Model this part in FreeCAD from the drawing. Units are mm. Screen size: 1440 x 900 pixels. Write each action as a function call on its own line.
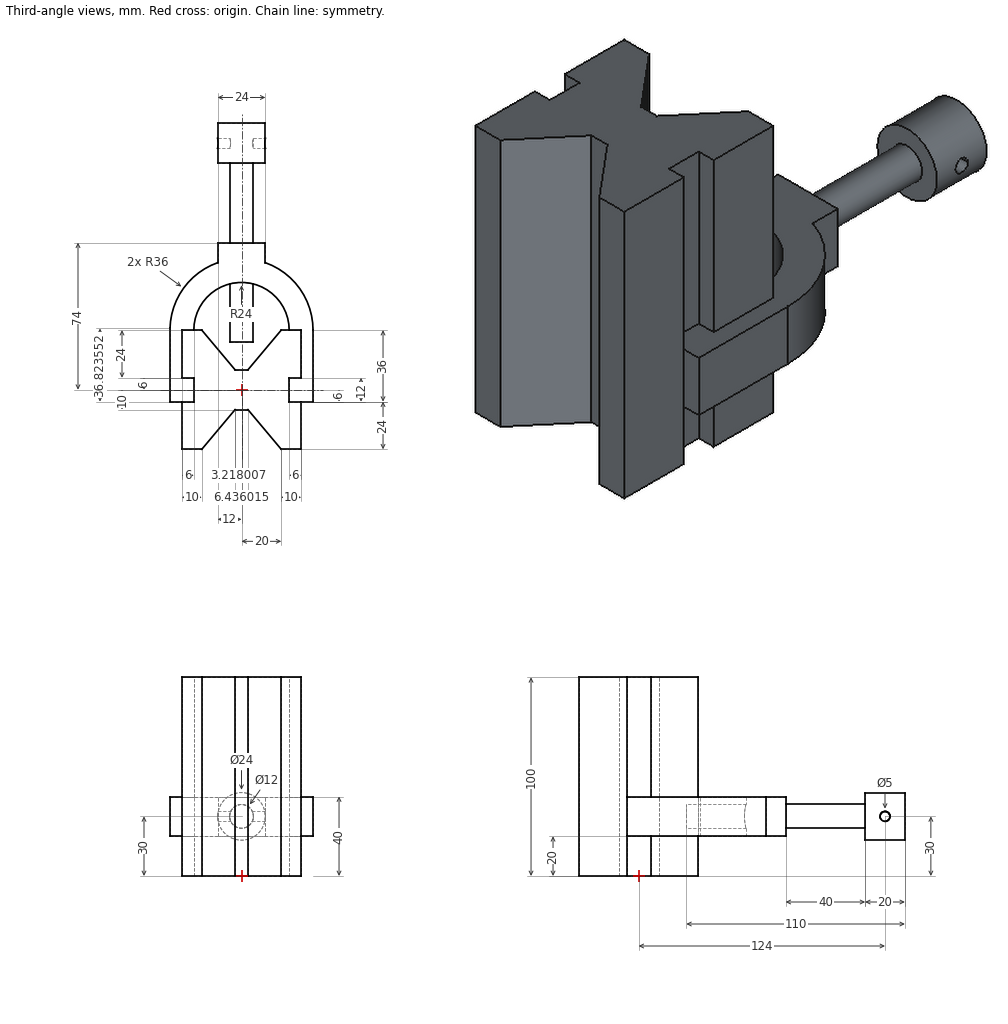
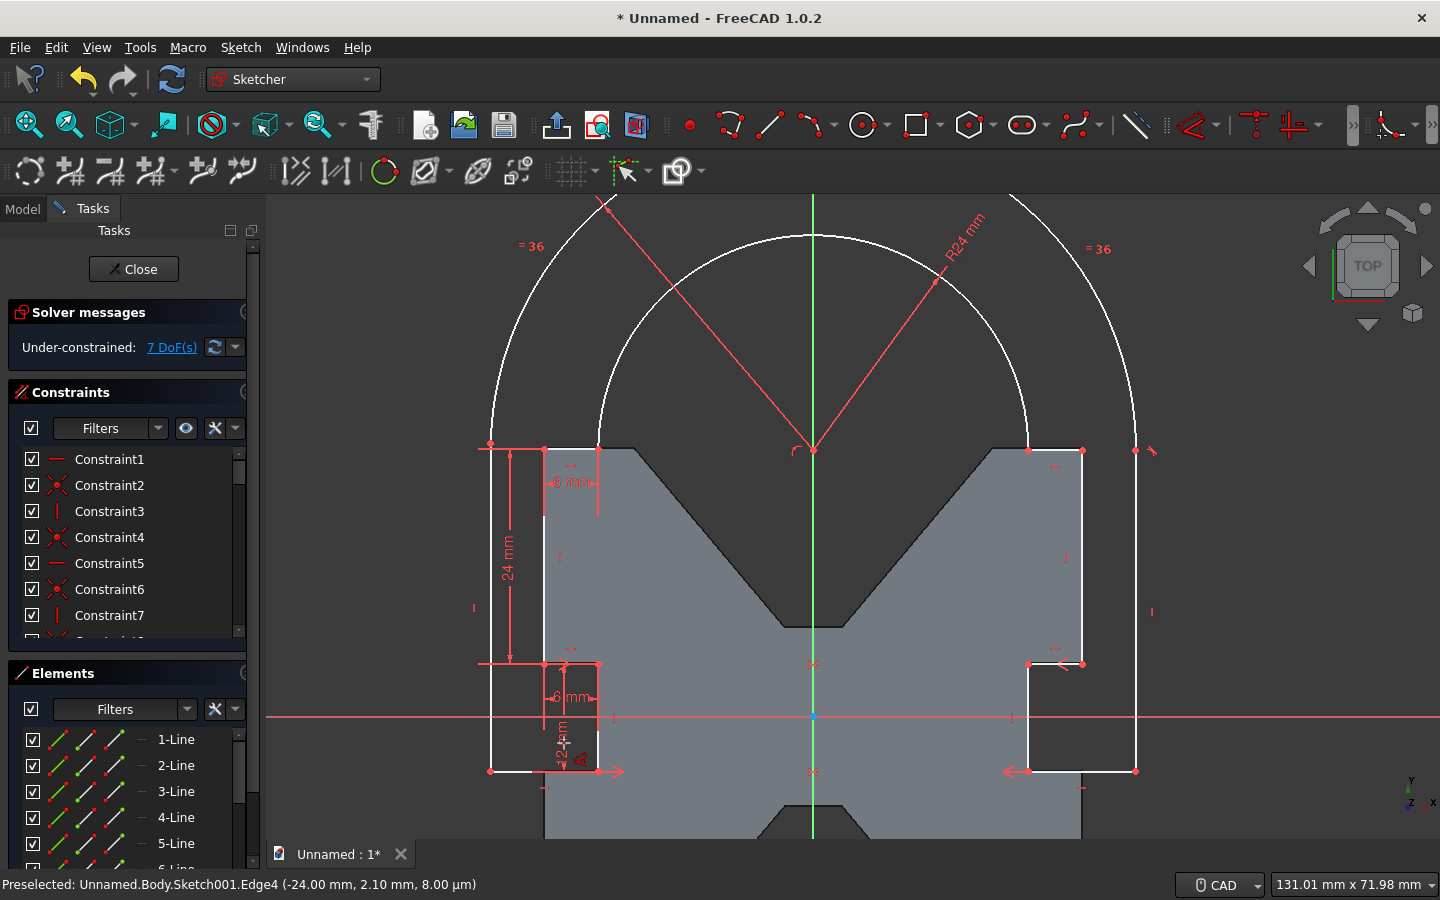
scroll(749, 643, down, 3)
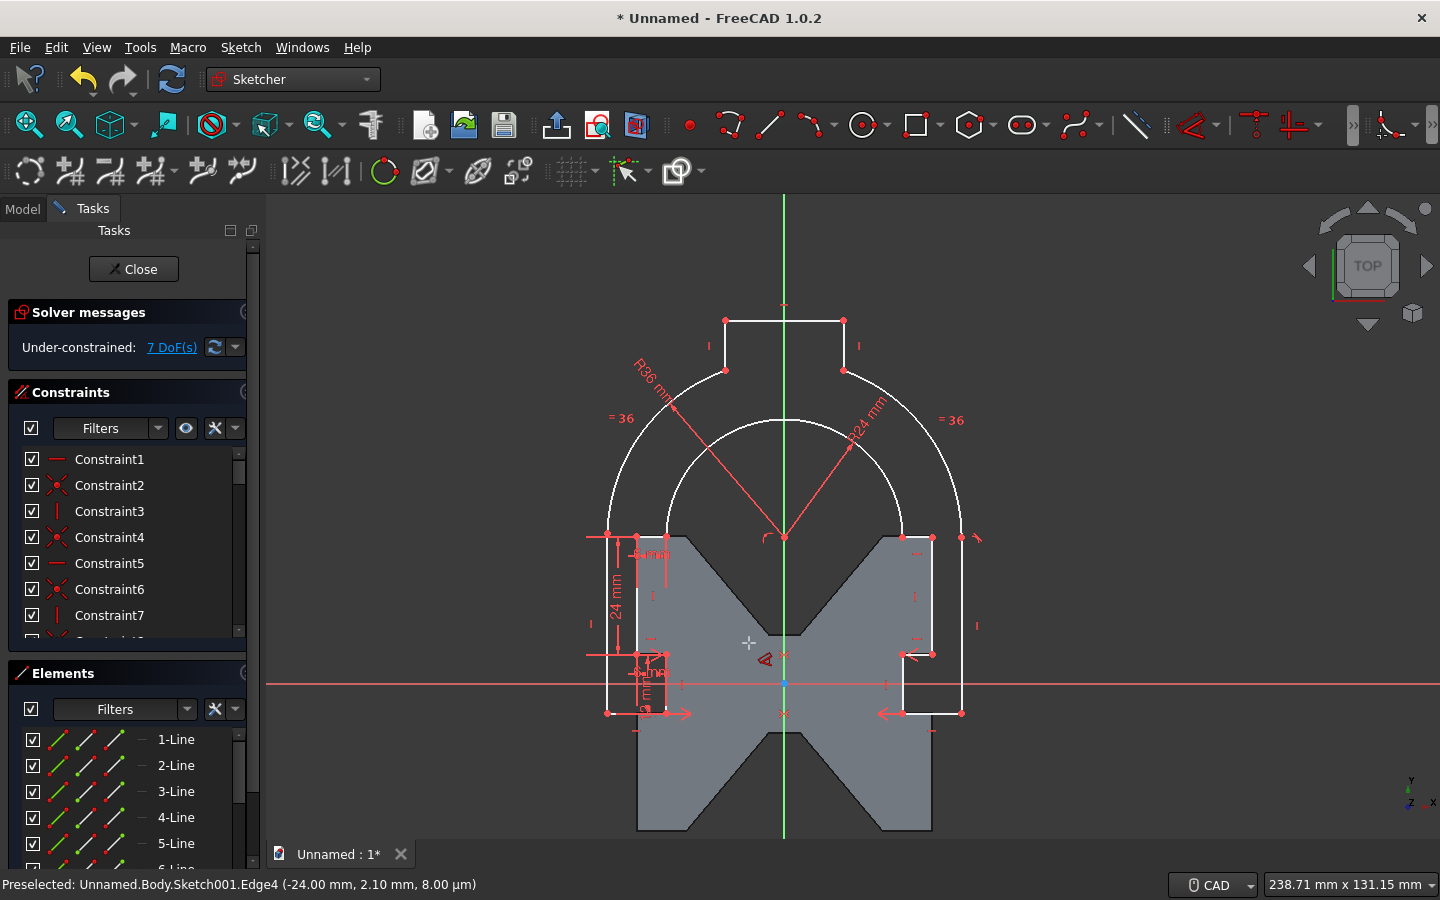
click(761, 321)
click(757, 287)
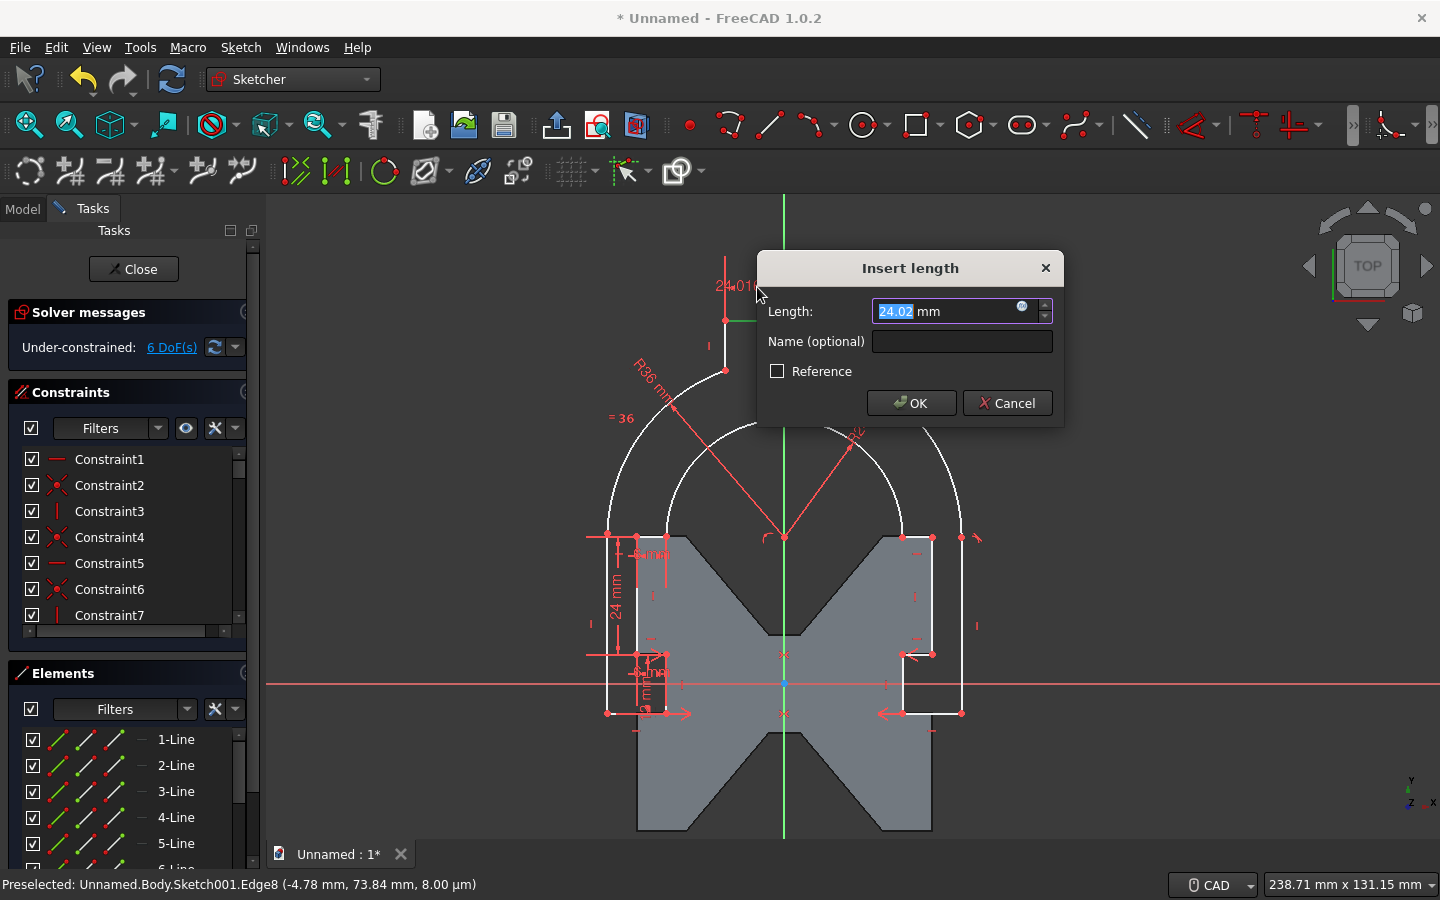
text(24)
key(Return)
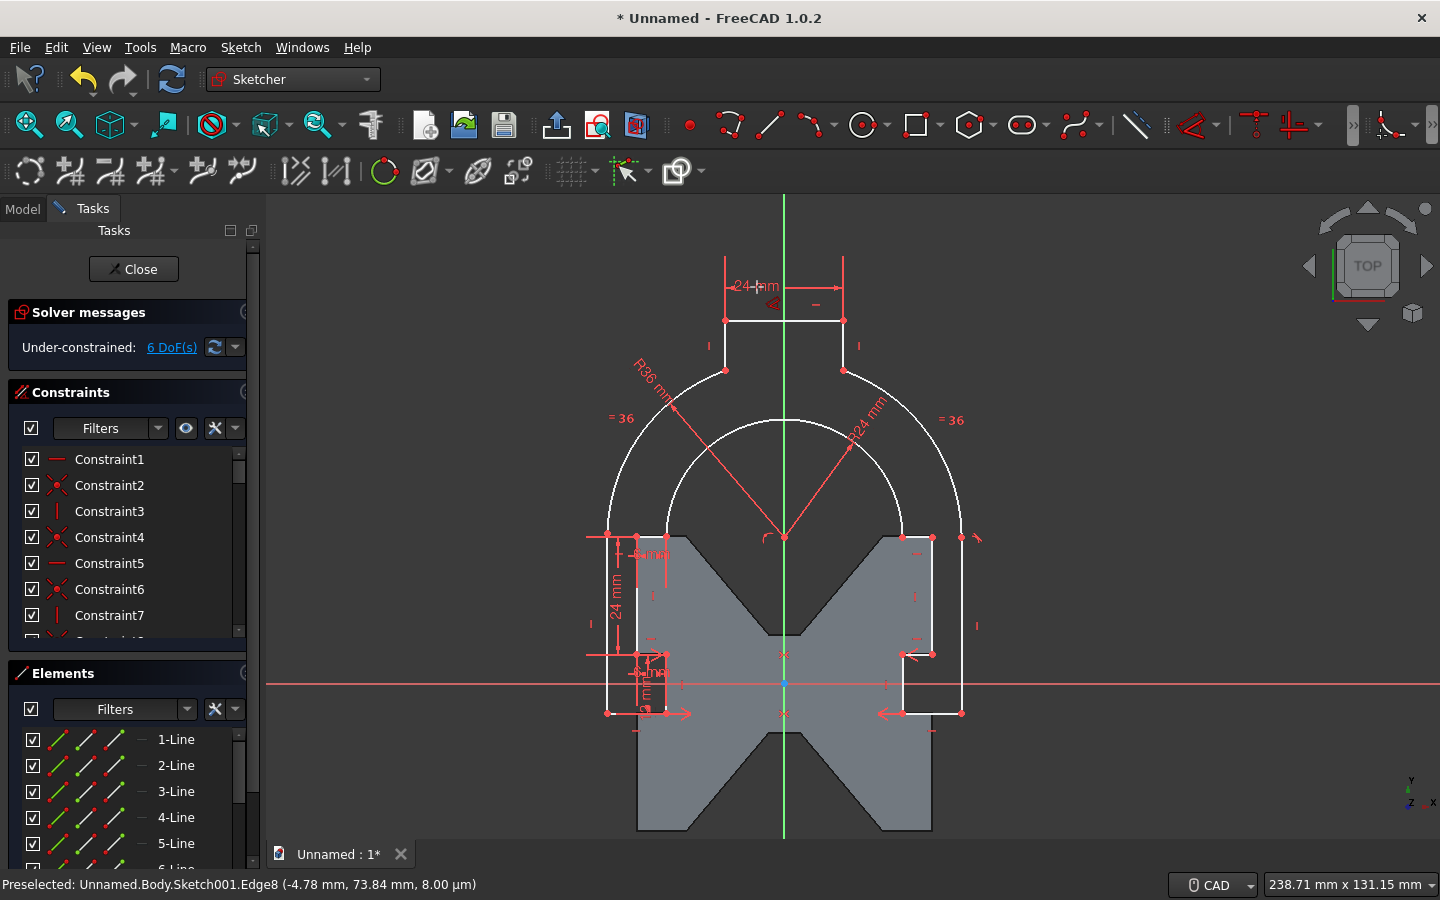
click(962, 590)
click(996, 626)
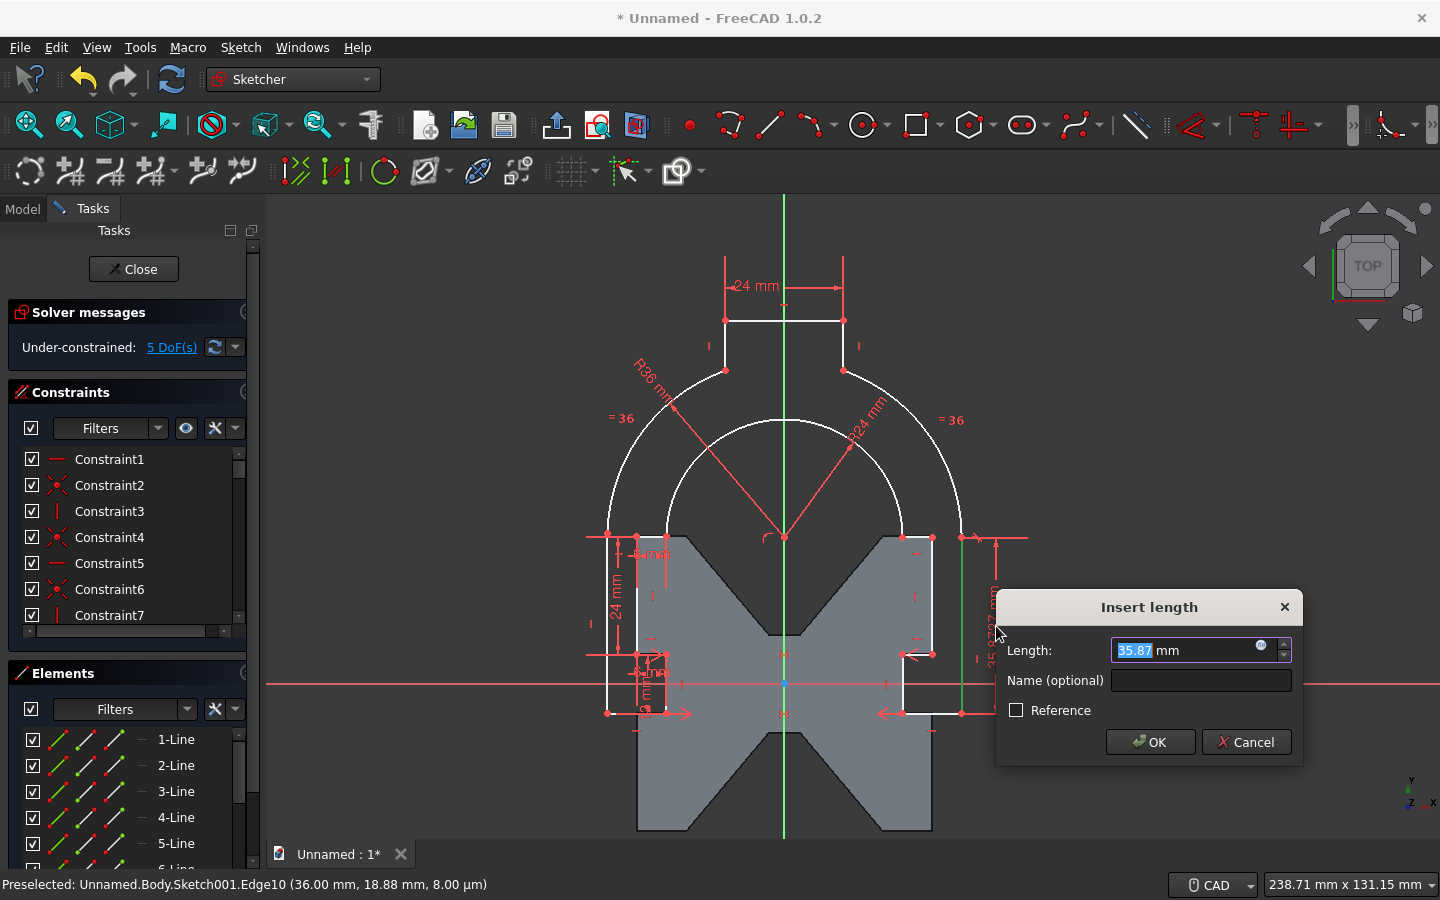
text(36)
key(Return)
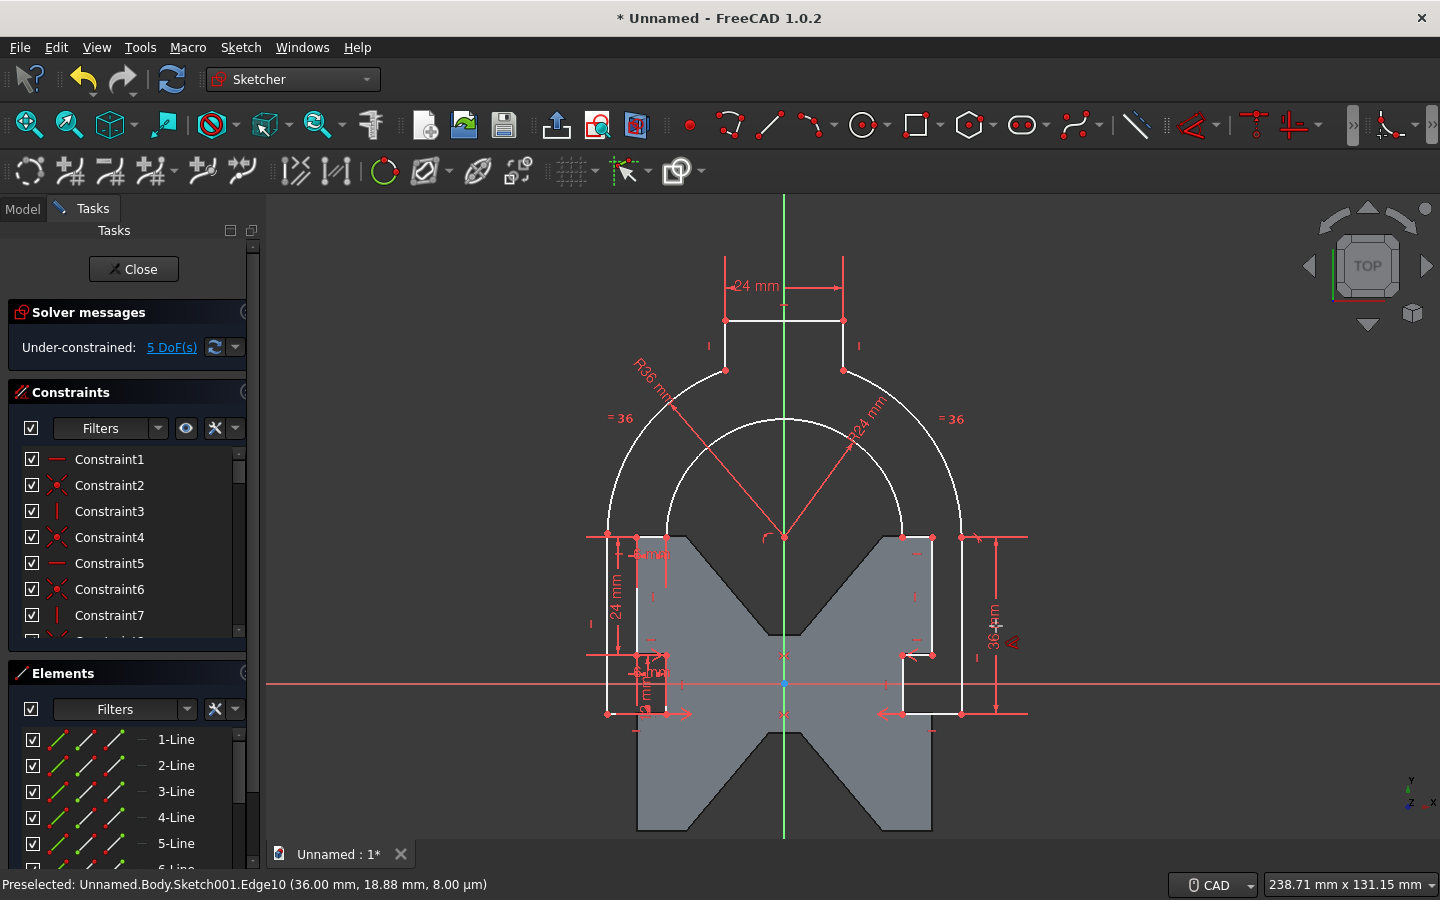
click(932, 620)
click(898, 596)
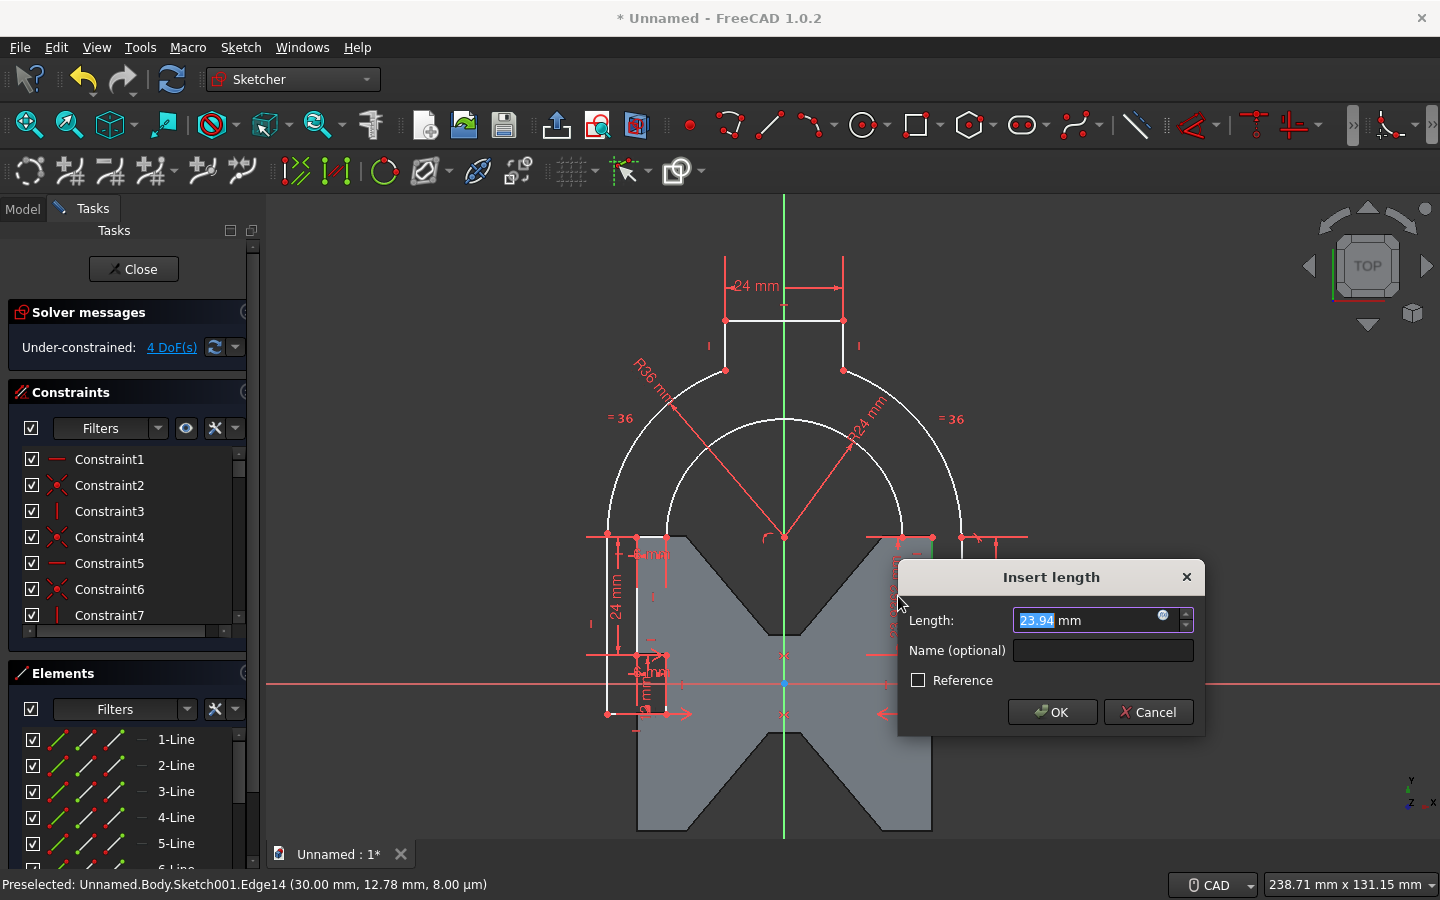
text(24)
key(Return)